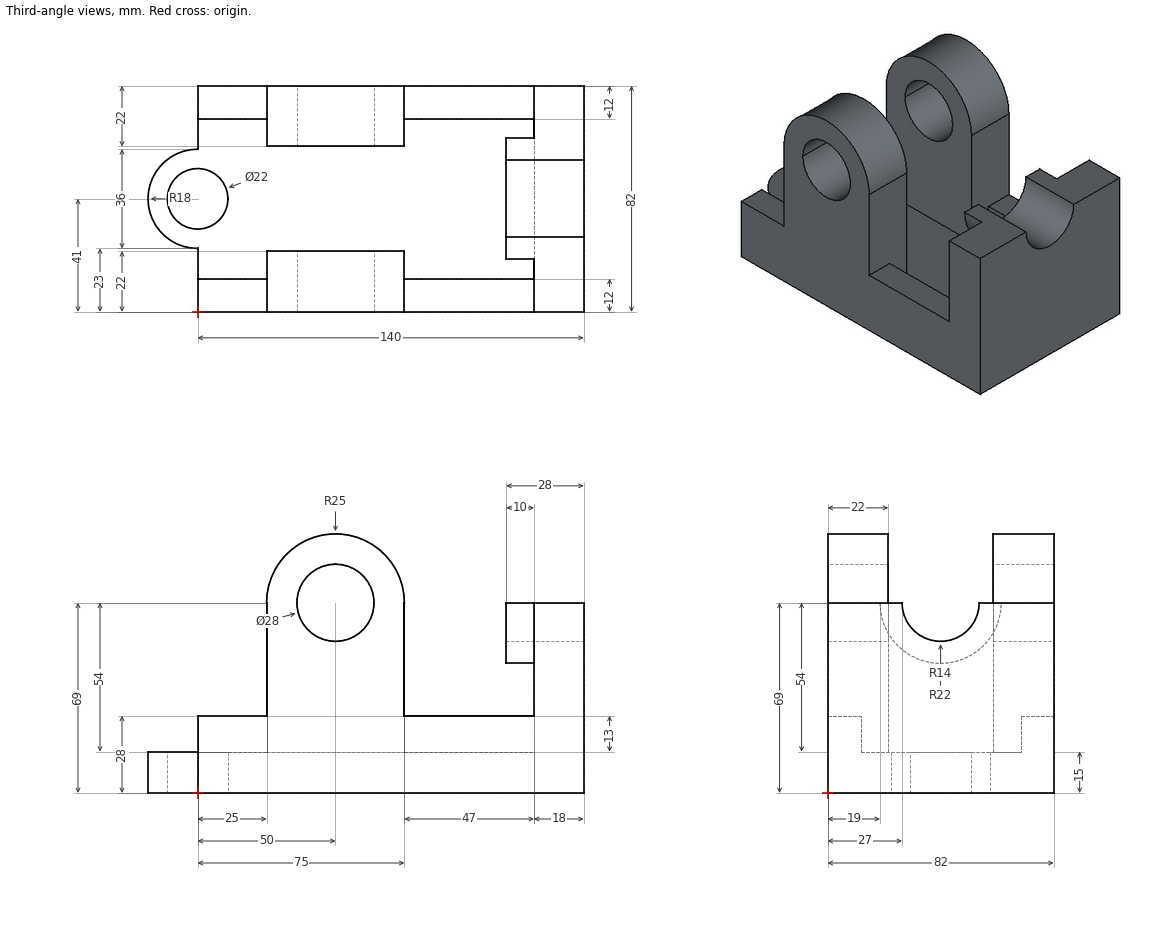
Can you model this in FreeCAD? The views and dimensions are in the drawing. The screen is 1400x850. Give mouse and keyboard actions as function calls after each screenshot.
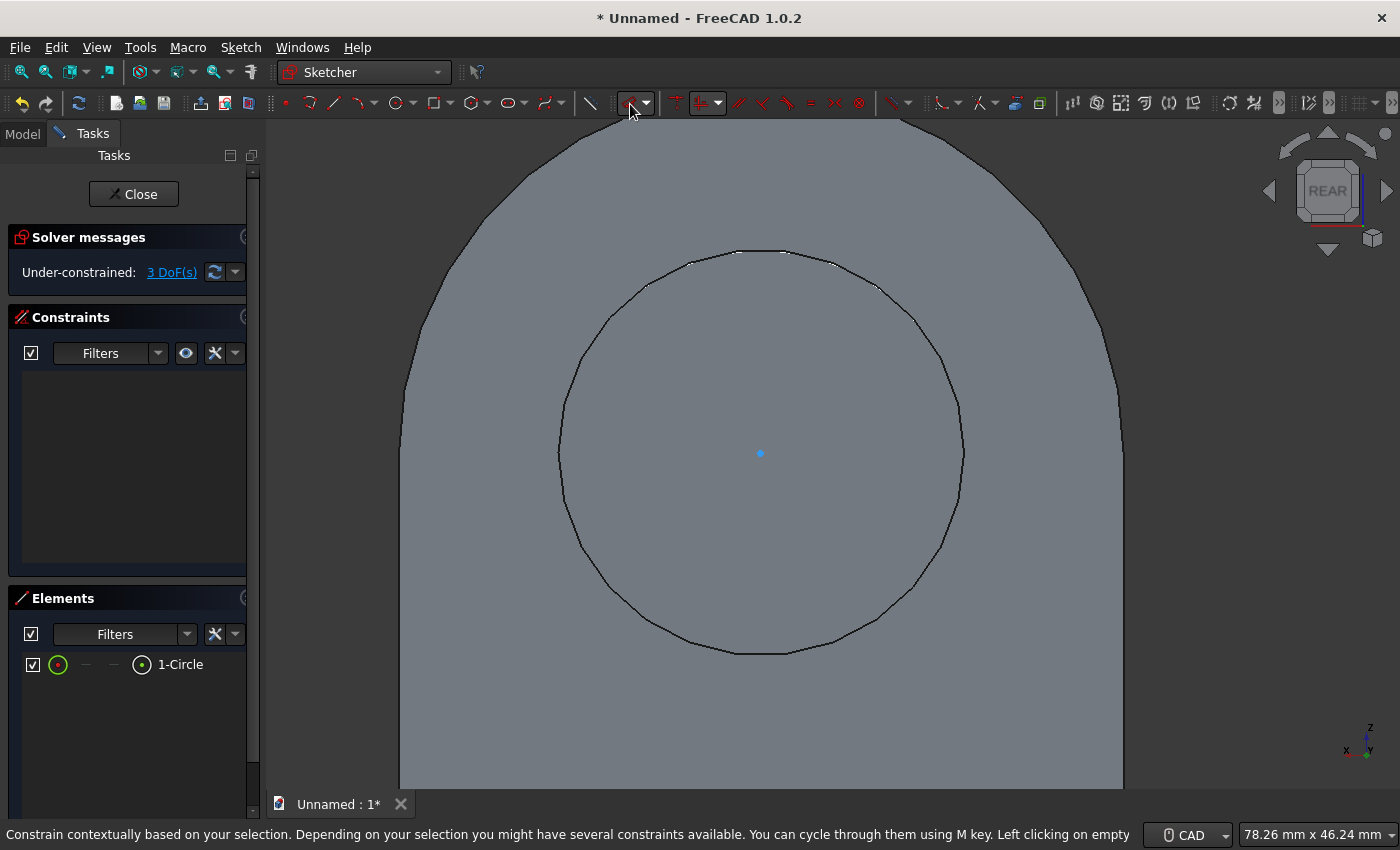
click(905, 310)
click(928, 287)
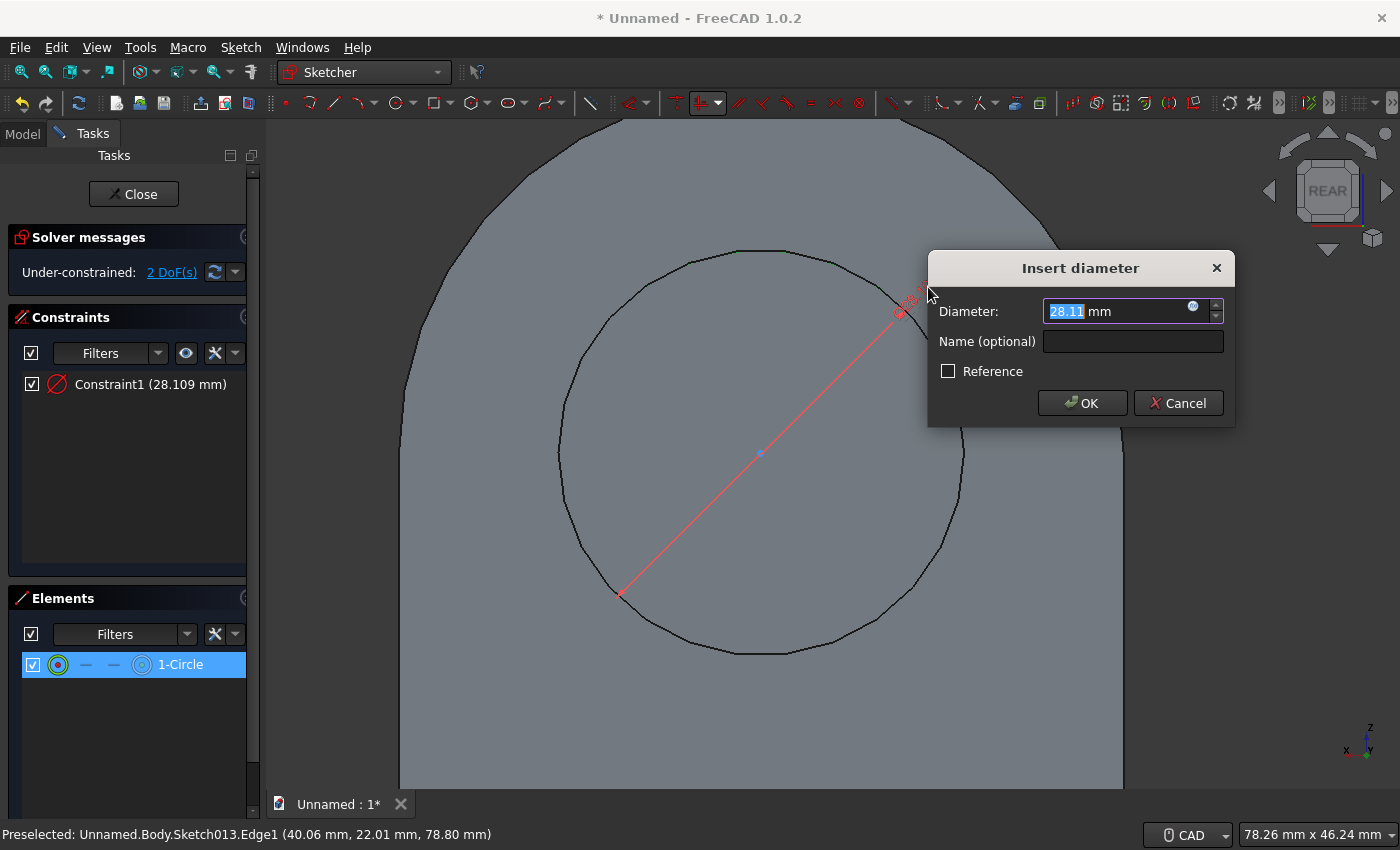
text(28)
key(Return)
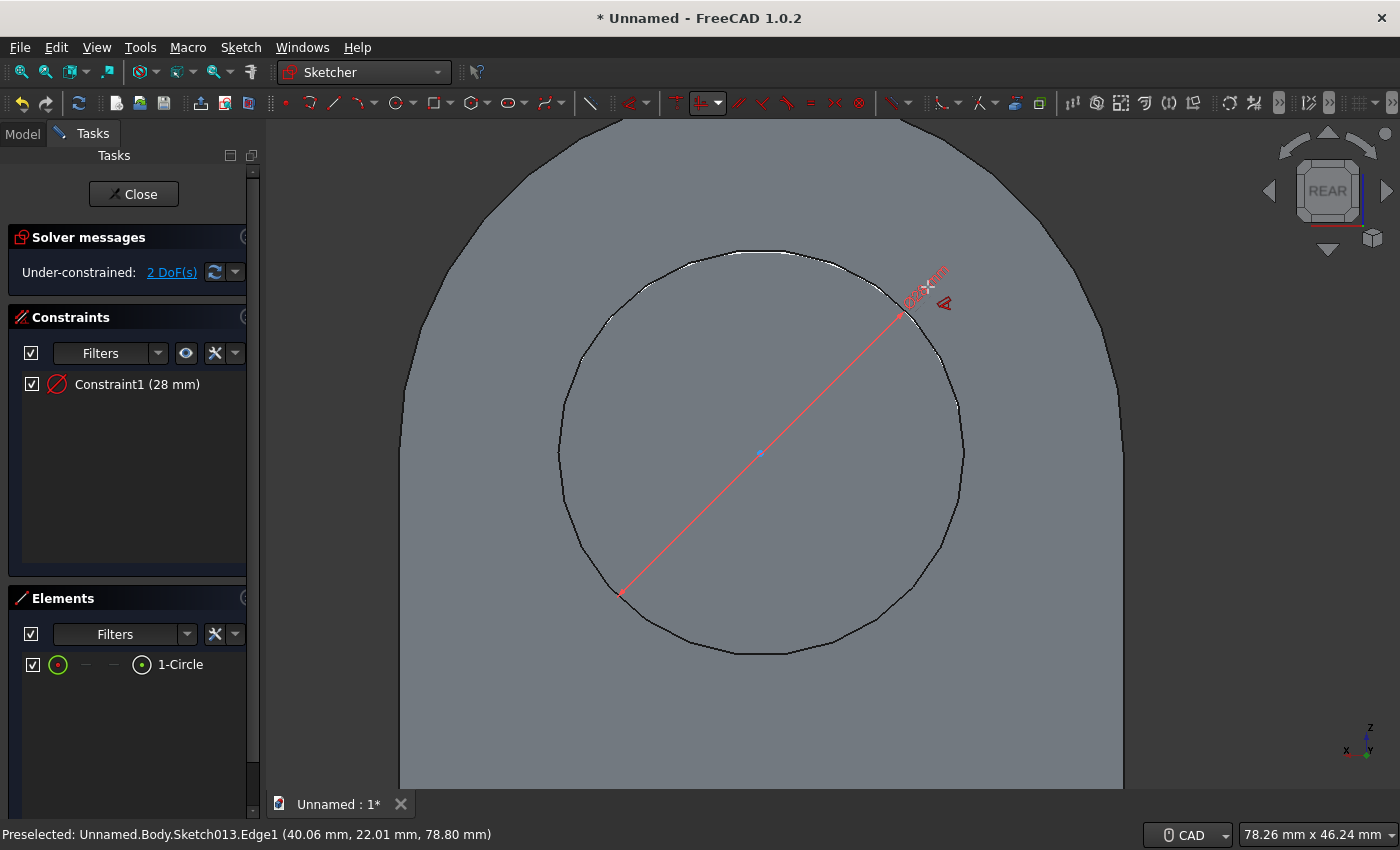
click(761, 454)
click(998, 420)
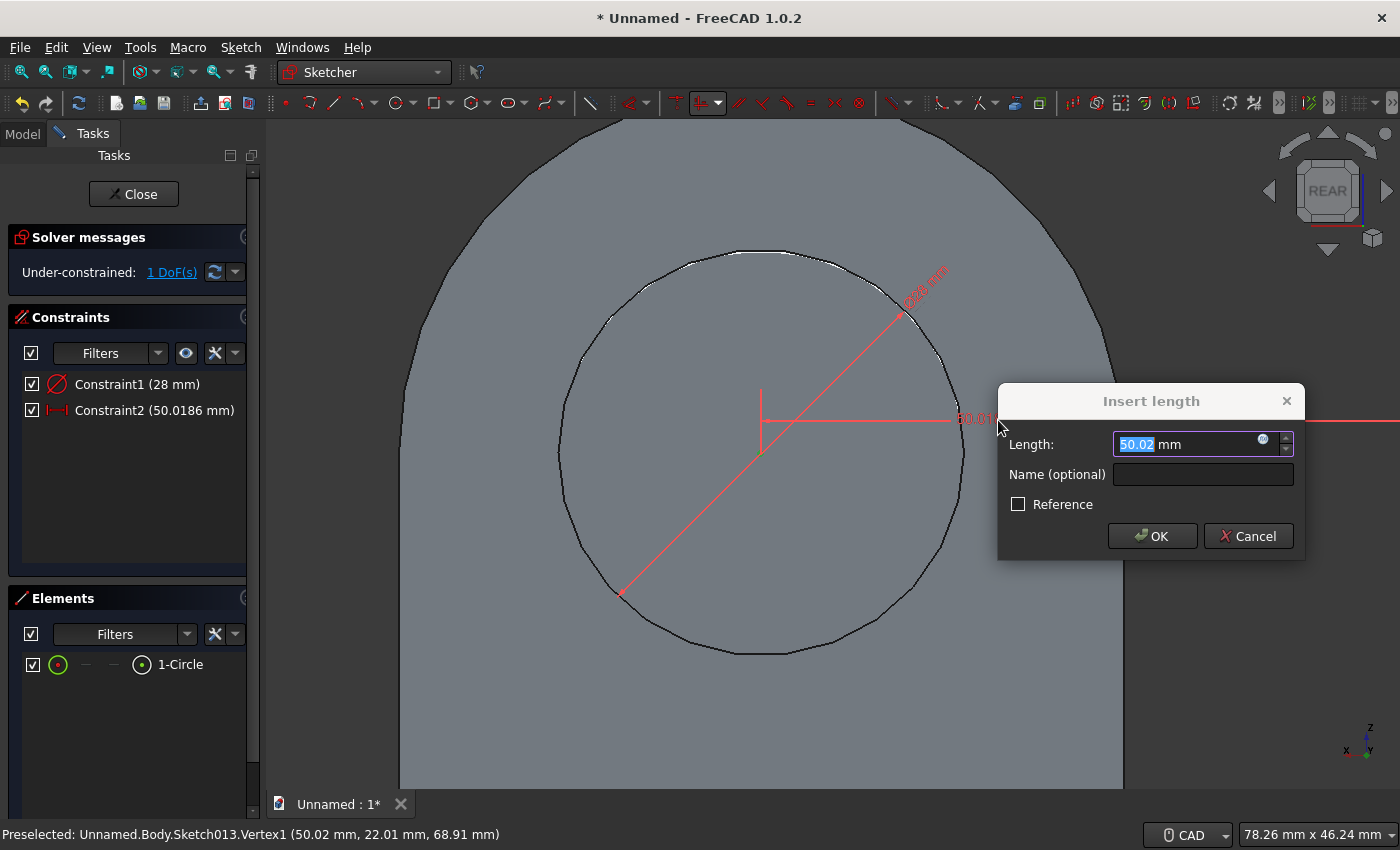
text(50)
key(Return)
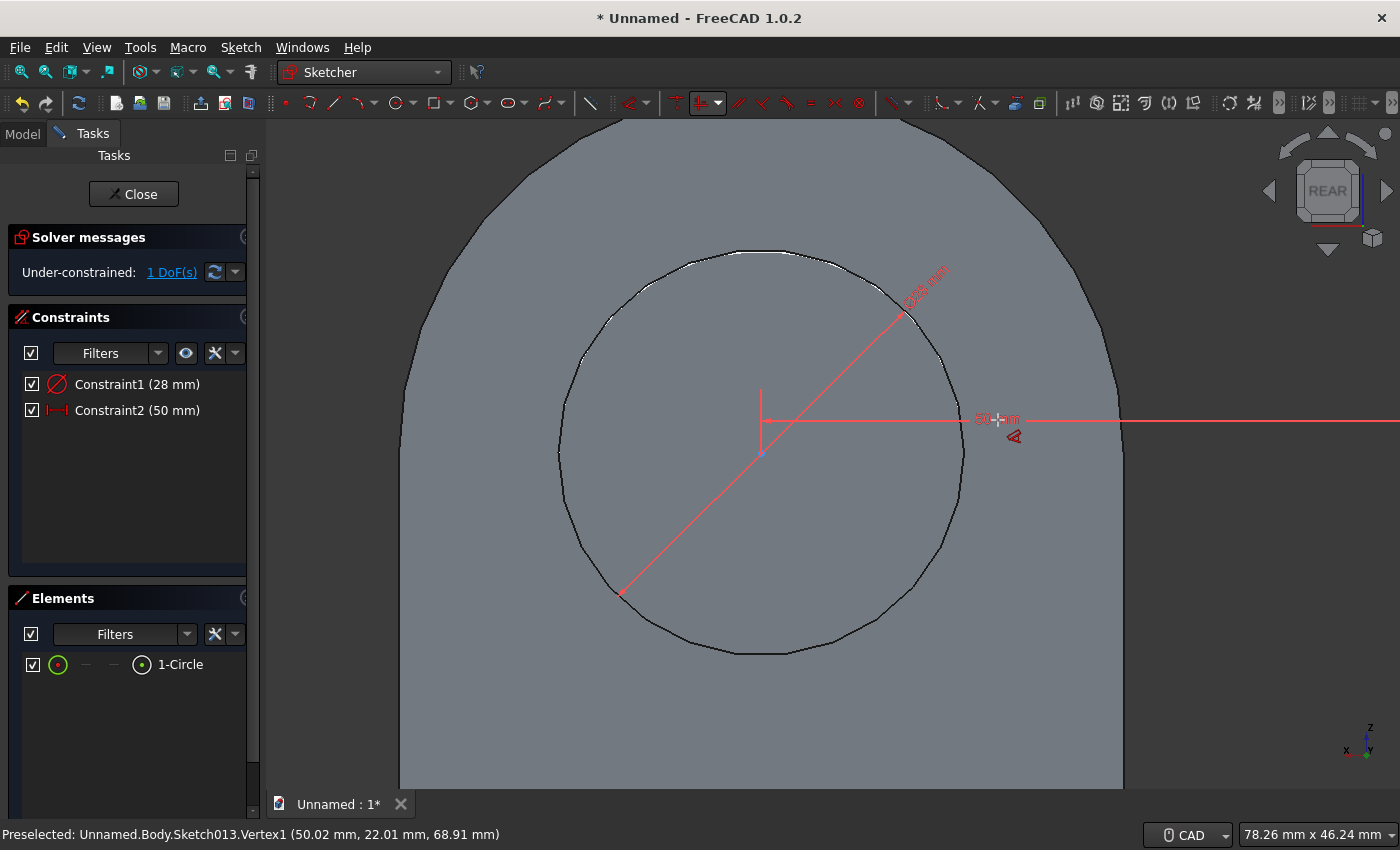
click(761, 454)
click(727, 608)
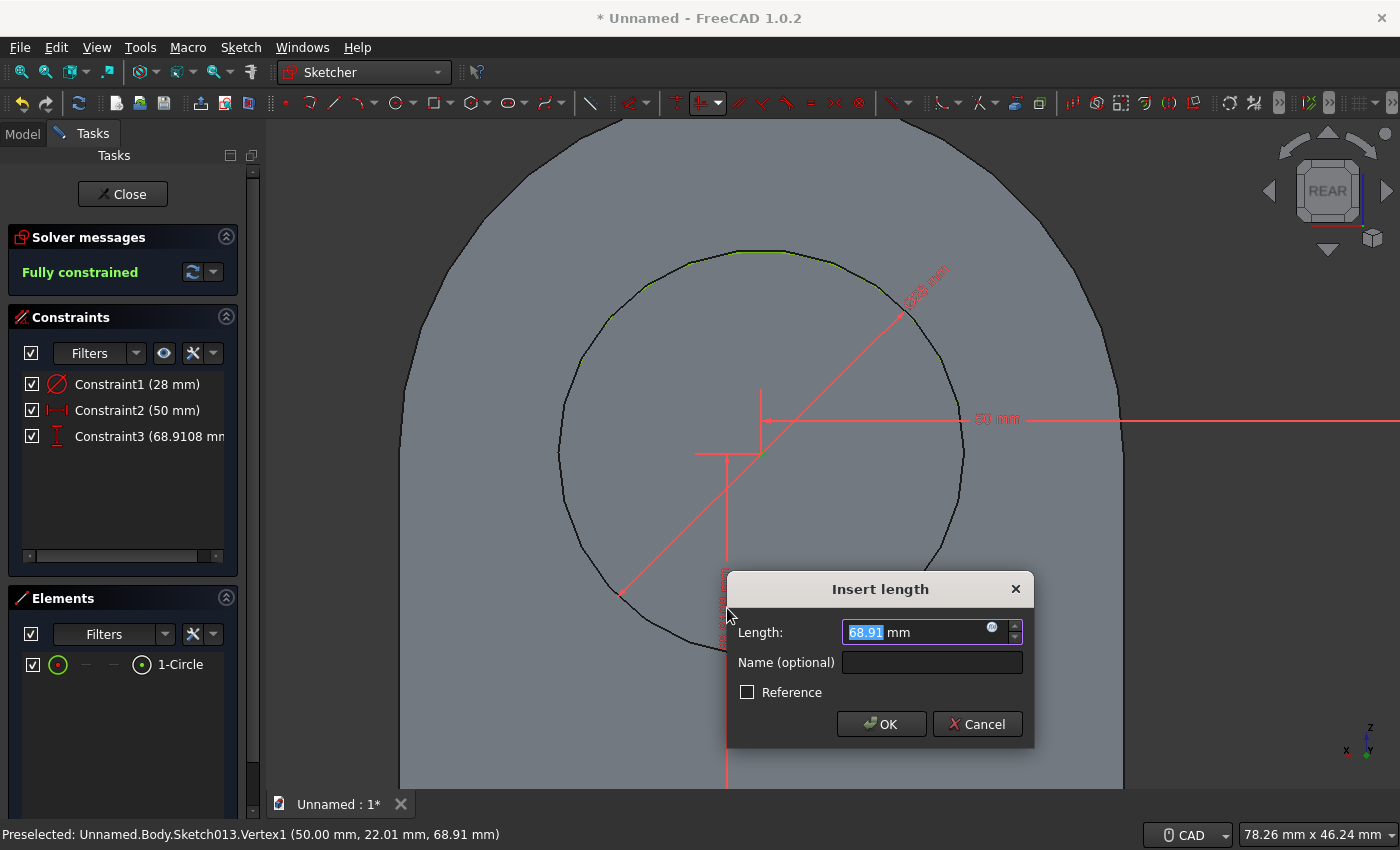
text(69)
key(Return)
key(Escape)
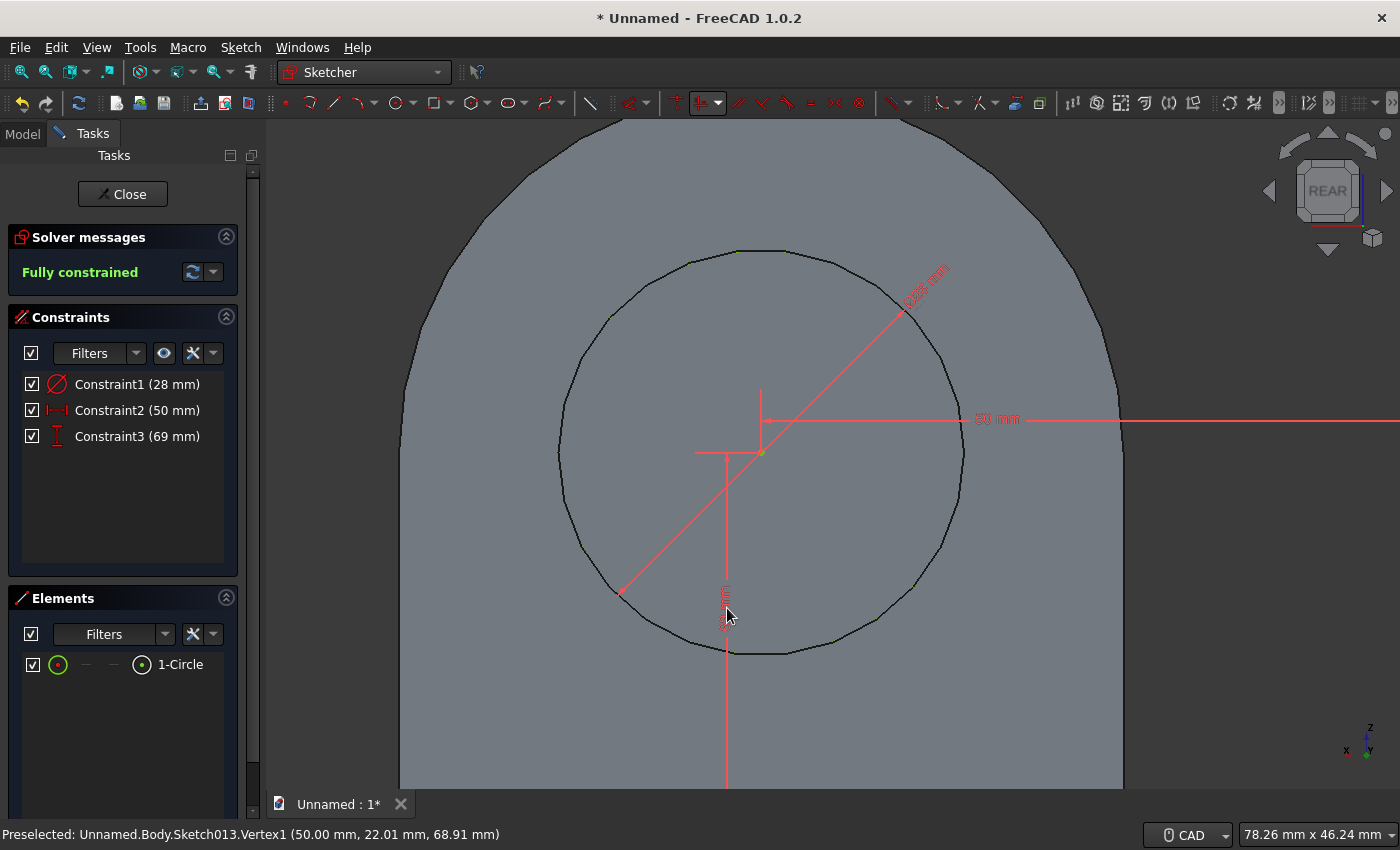
click(123, 194)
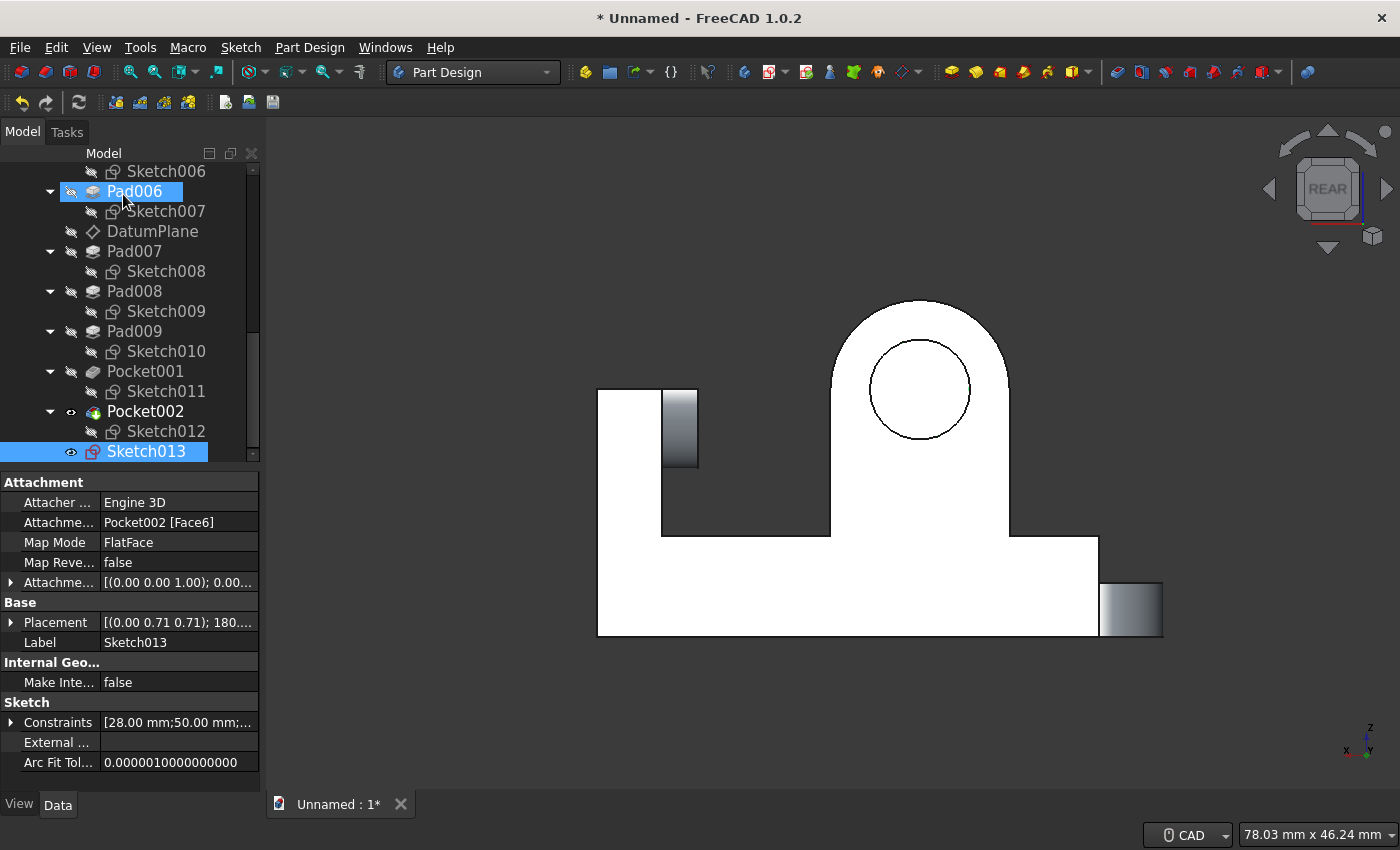
click(1118, 72)